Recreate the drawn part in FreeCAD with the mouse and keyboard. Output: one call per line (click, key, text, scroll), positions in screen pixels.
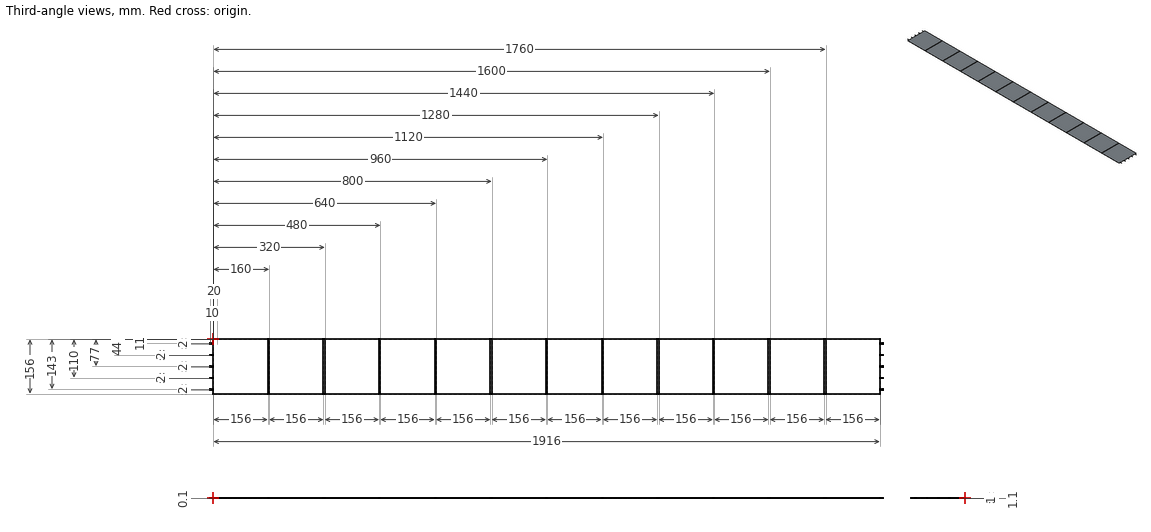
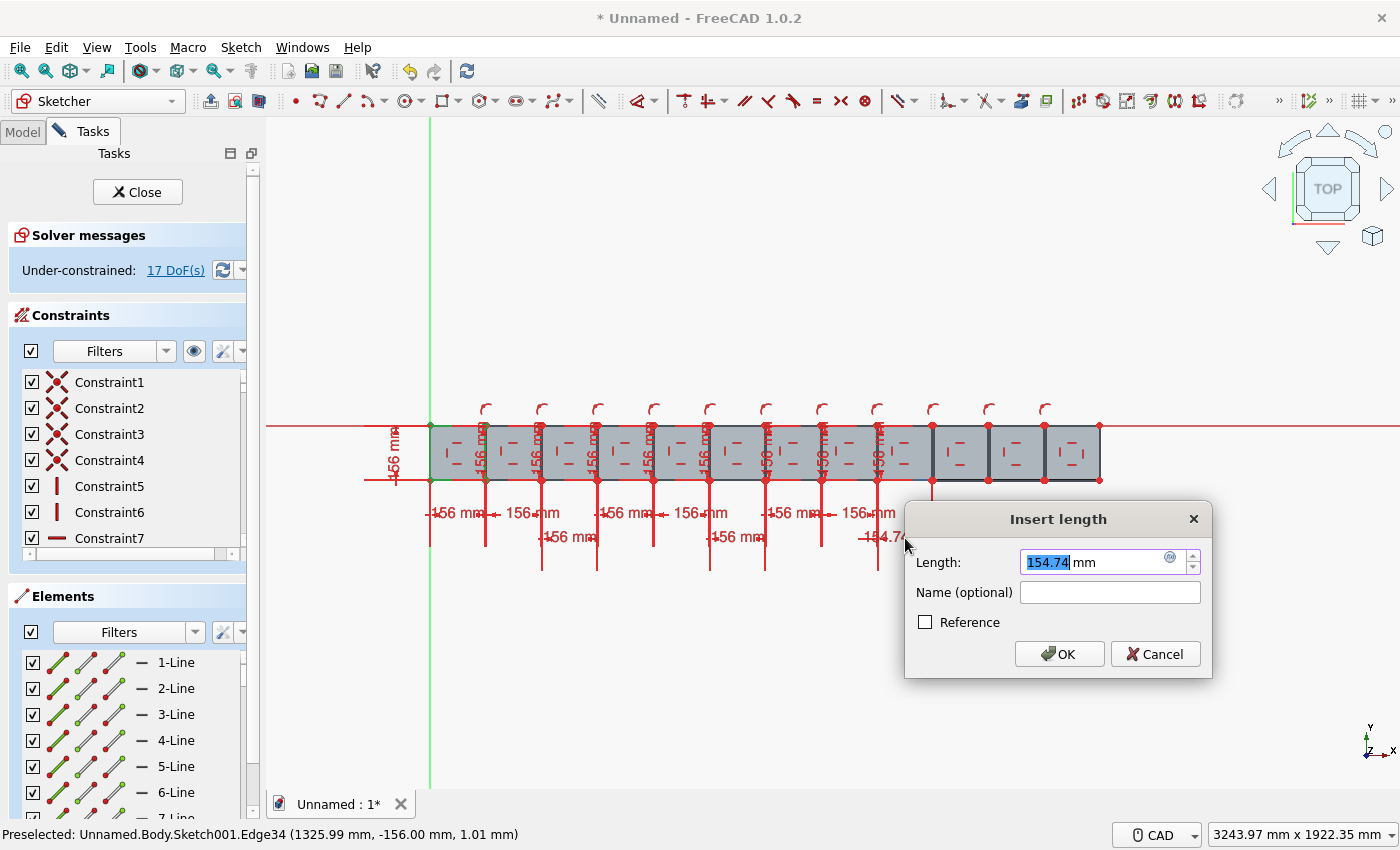
text(156)
key(Return)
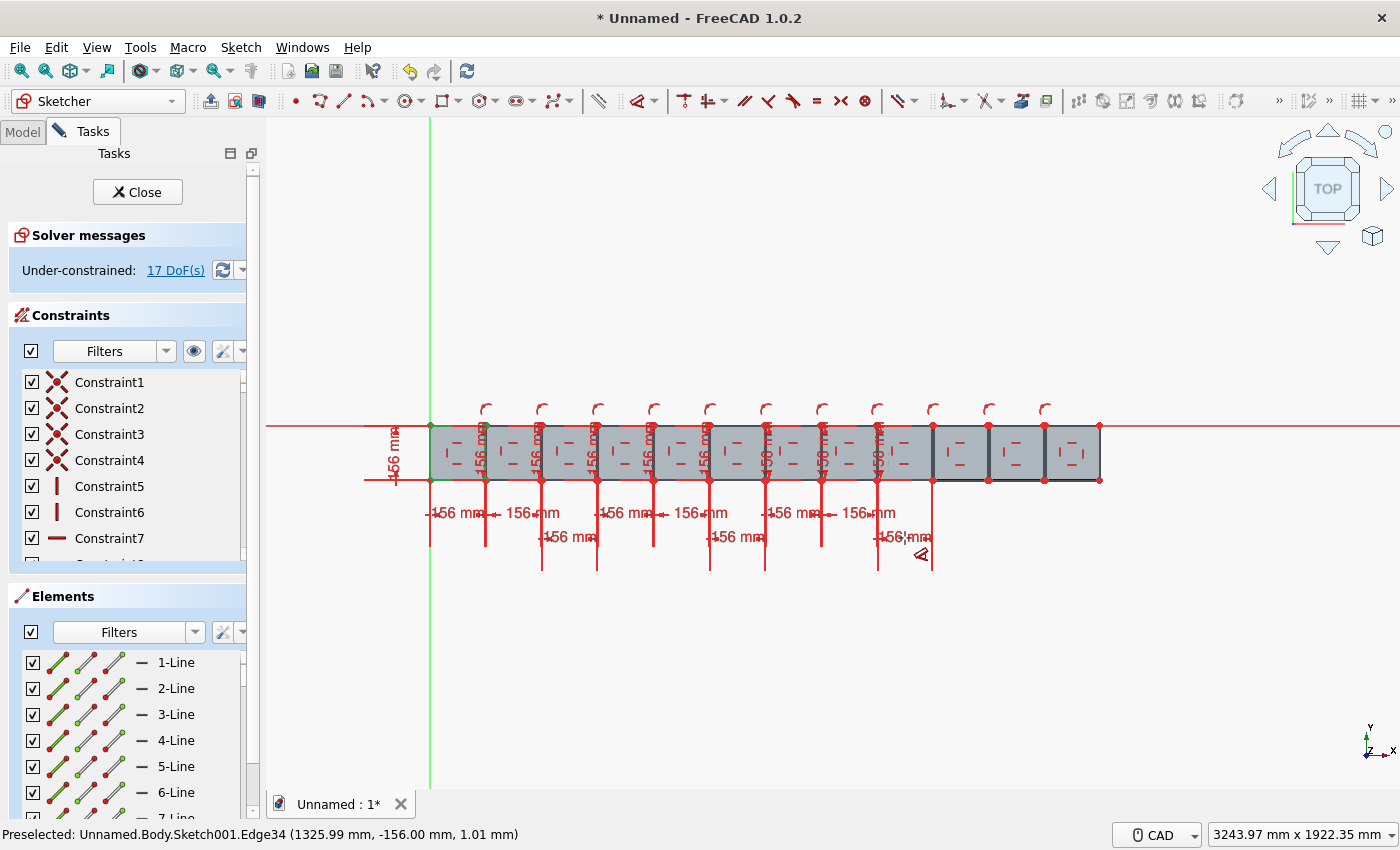
scroll(934, 442, up, 11)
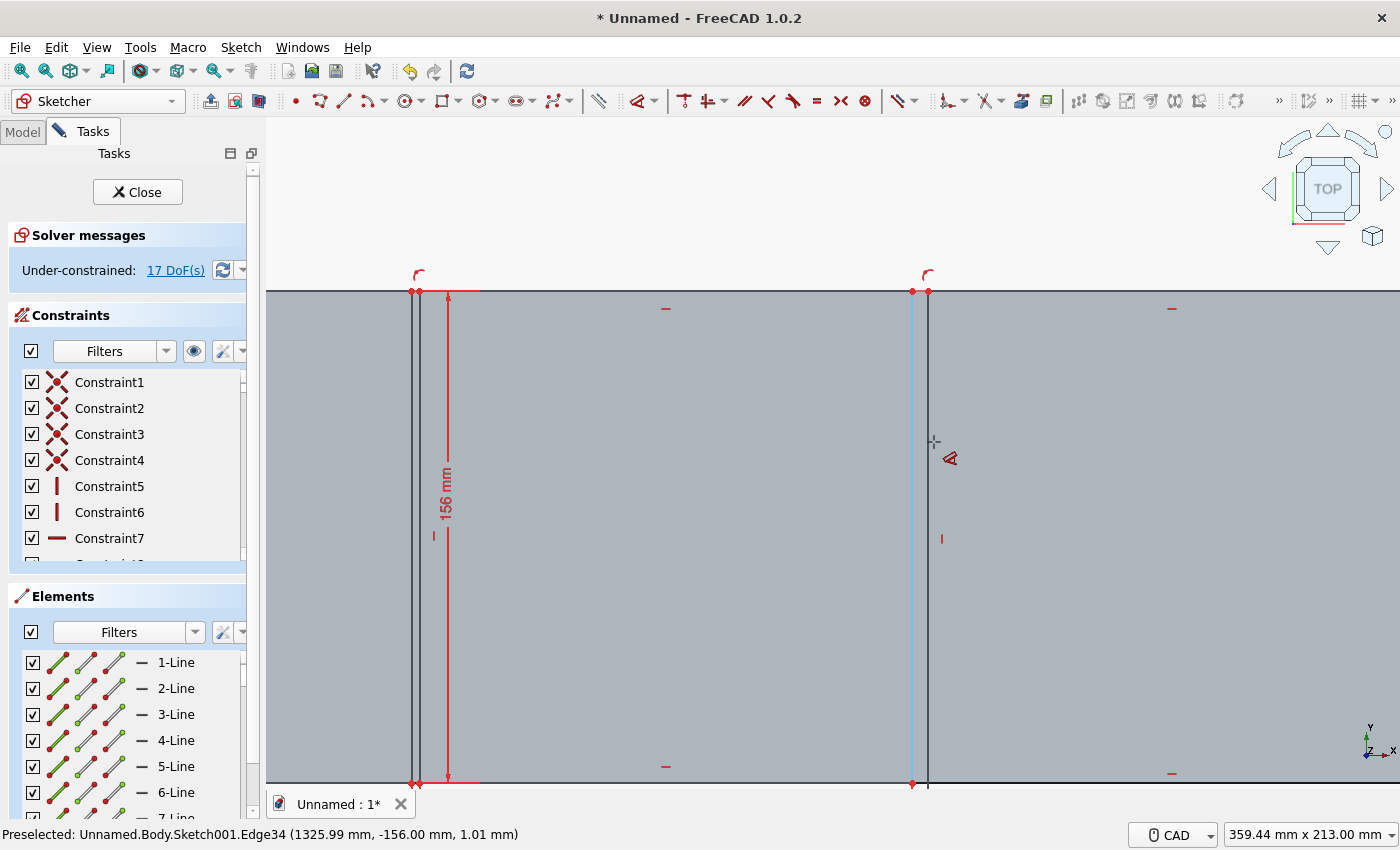
click(928, 441)
click(962, 526)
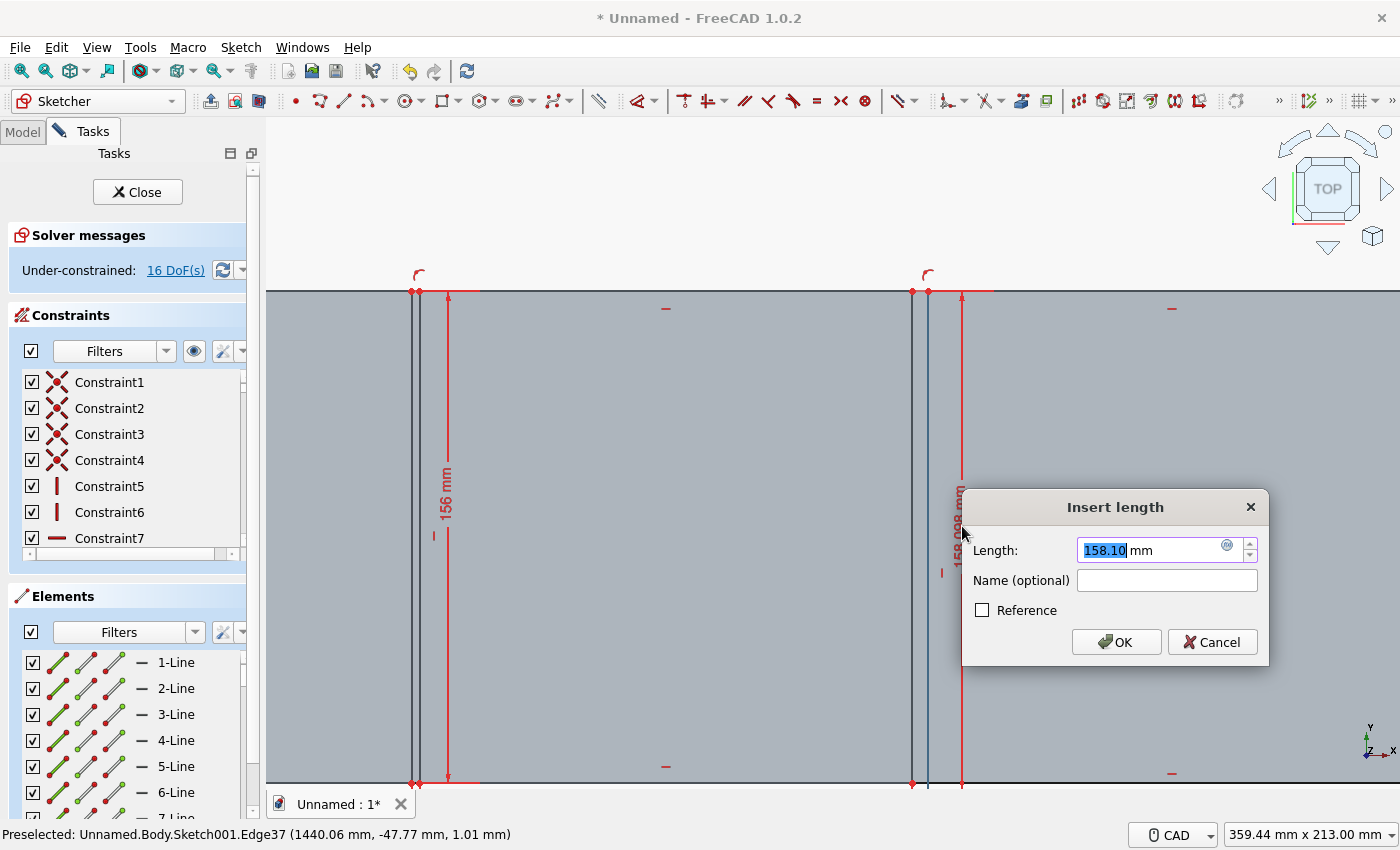
text(156)
key(Return)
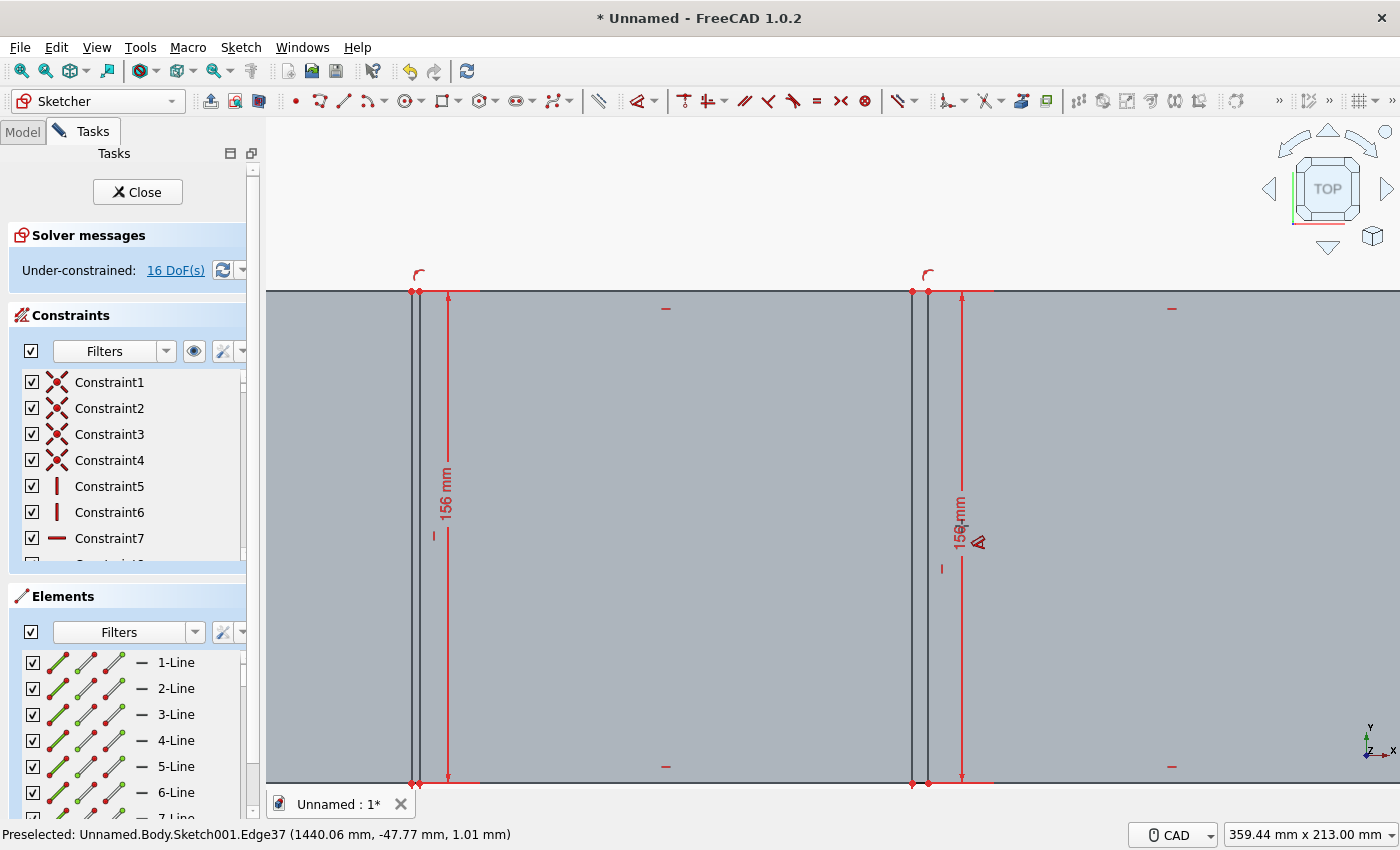
scroll(934, 442, down, 11)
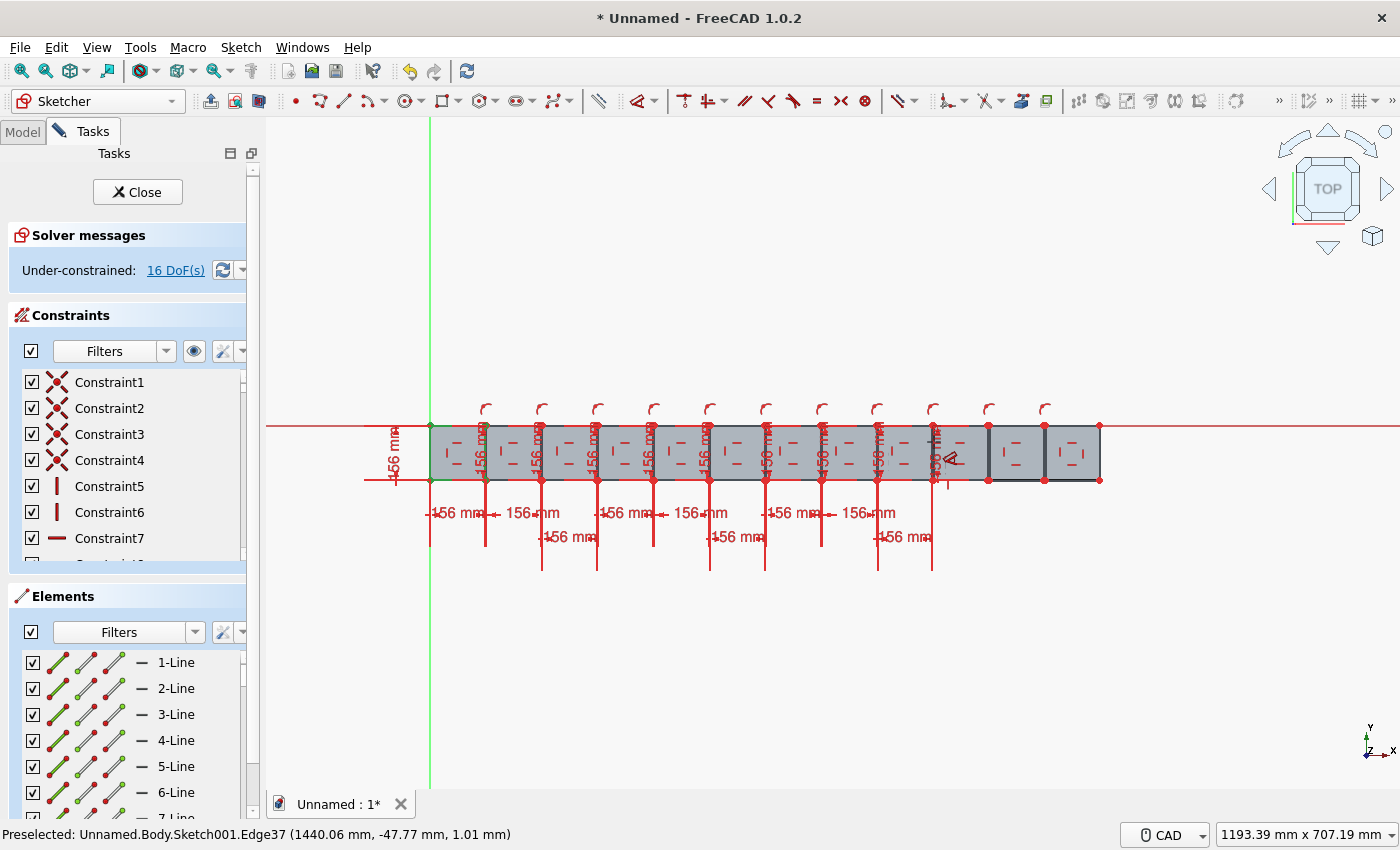
click(950, 480)
click(961, 514)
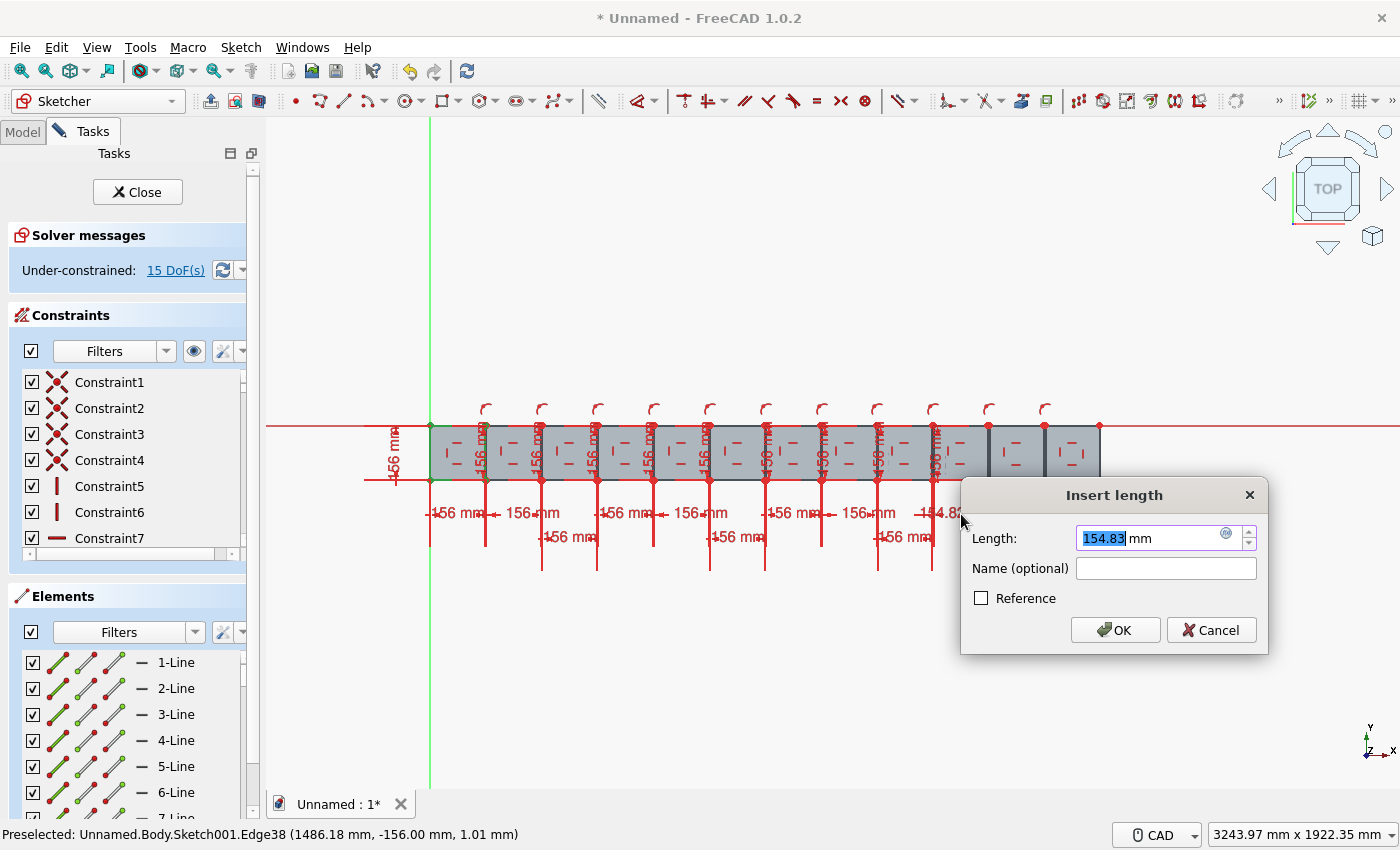
text(156)
key(Return)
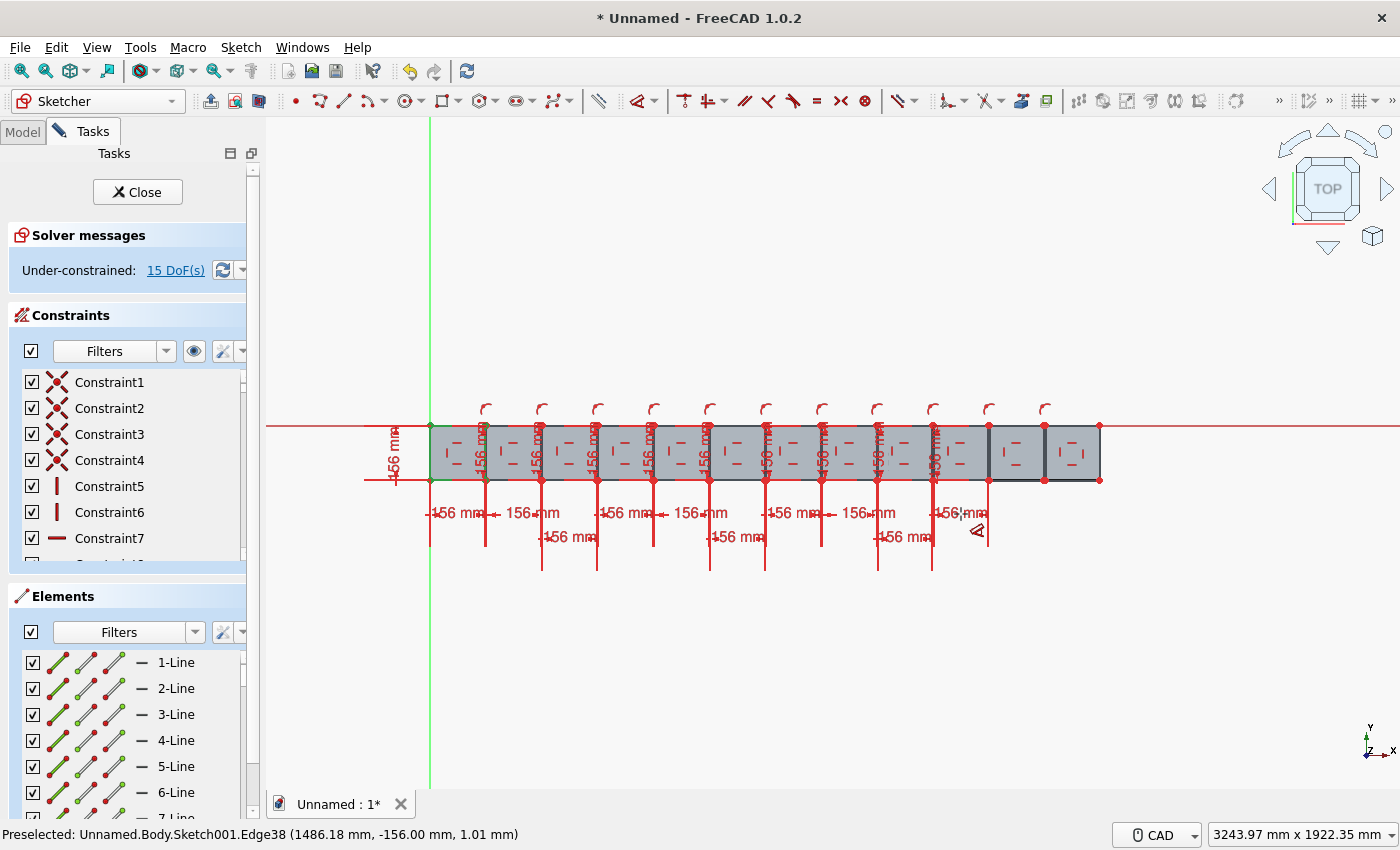
scroll(990, 442, up, 11)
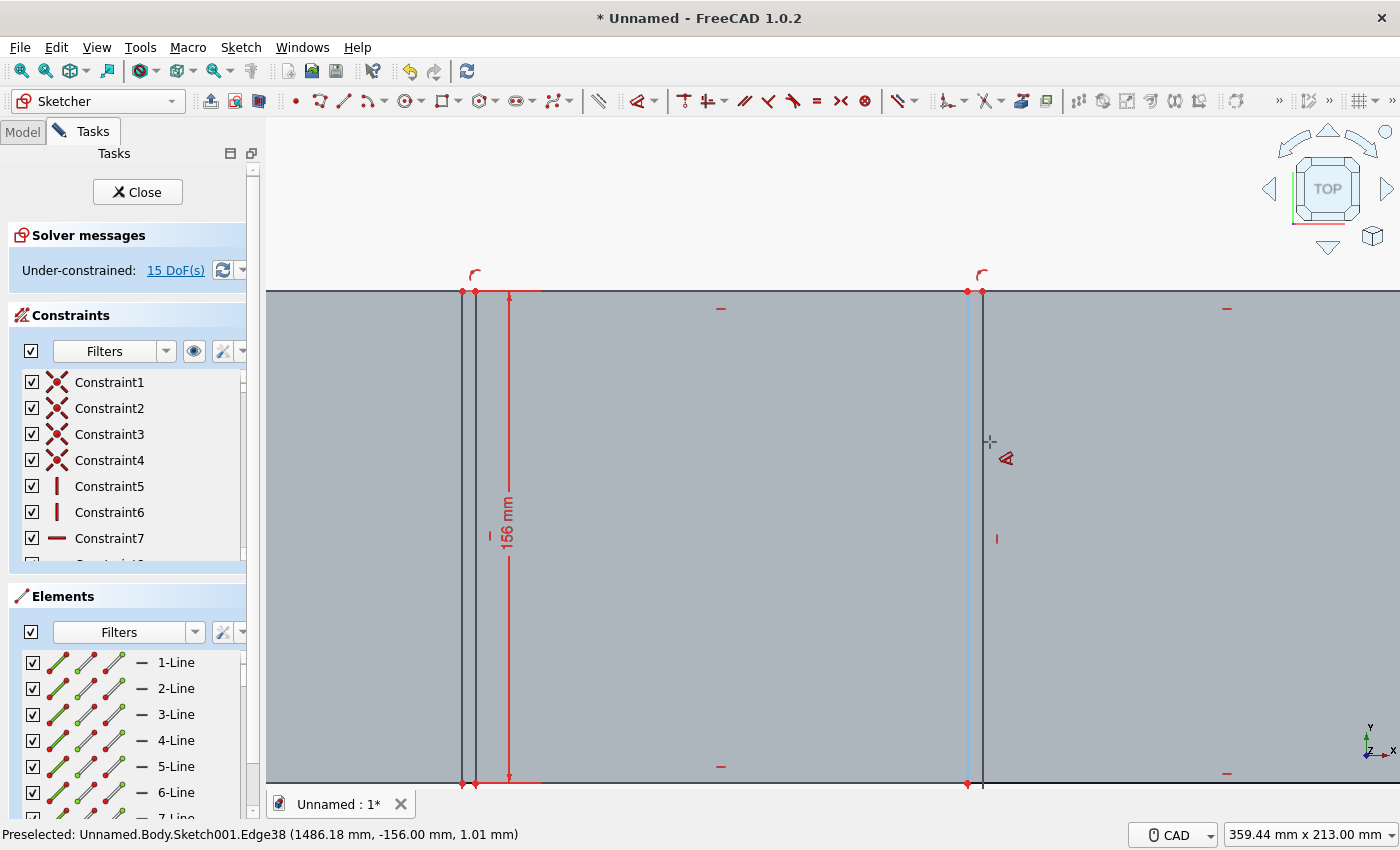
click(983, 441)
click(1017, 526)